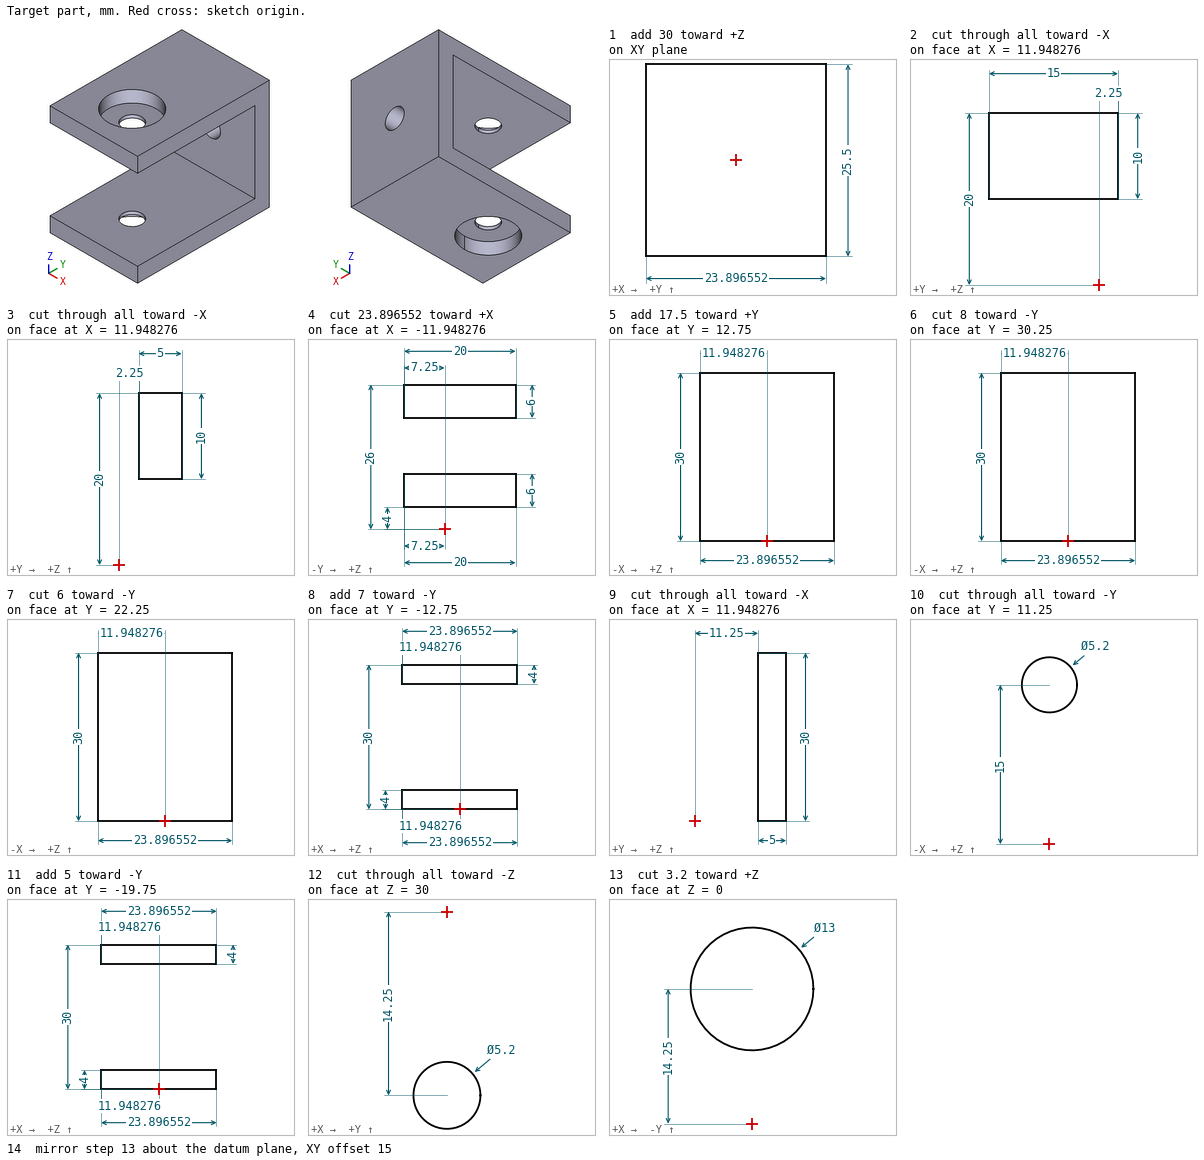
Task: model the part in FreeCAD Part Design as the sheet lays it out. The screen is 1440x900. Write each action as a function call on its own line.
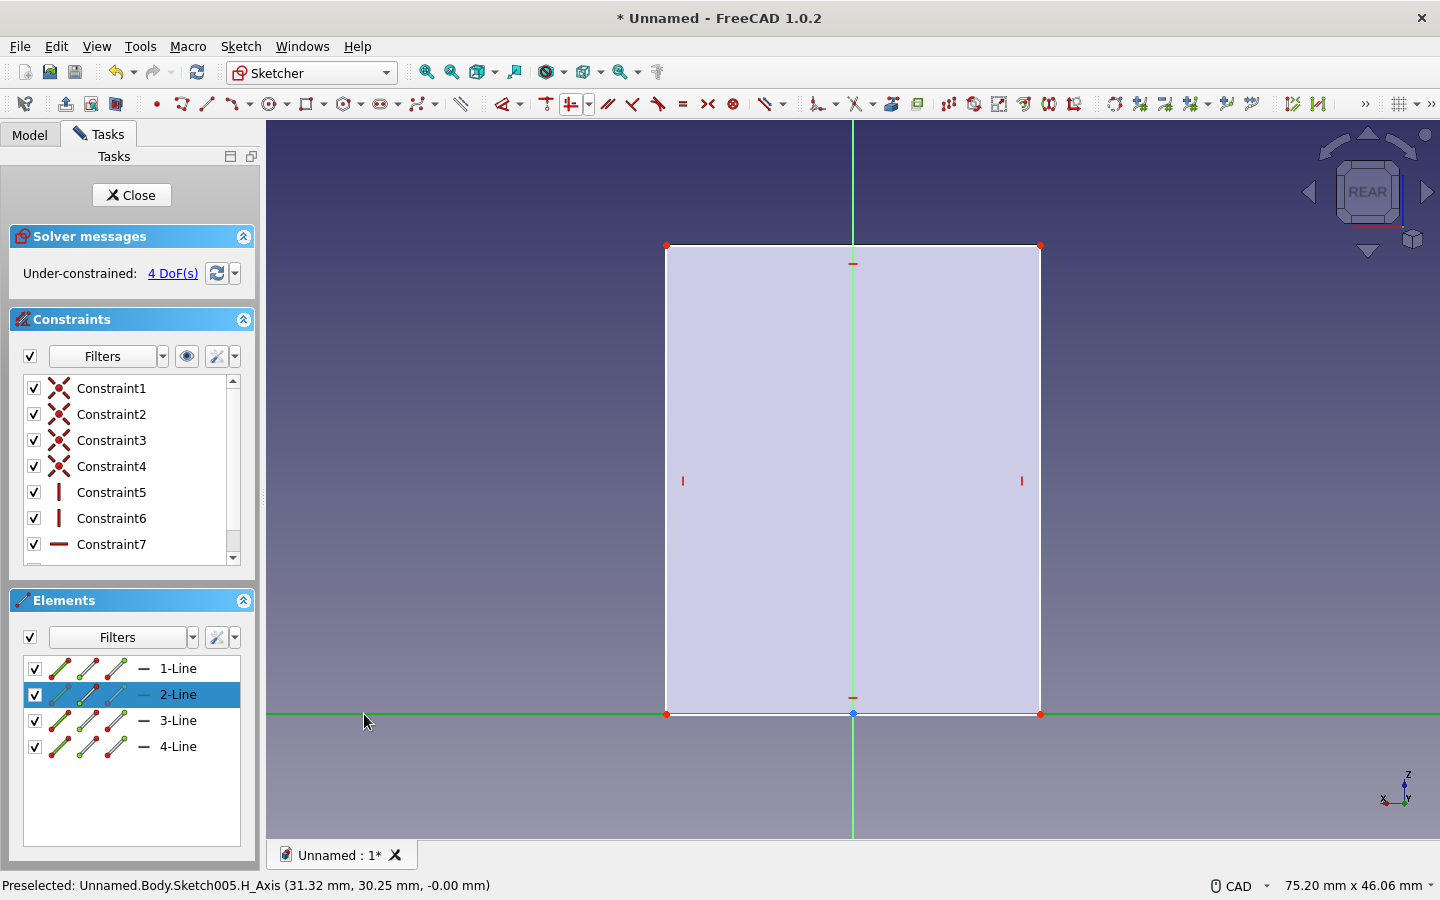
key(c)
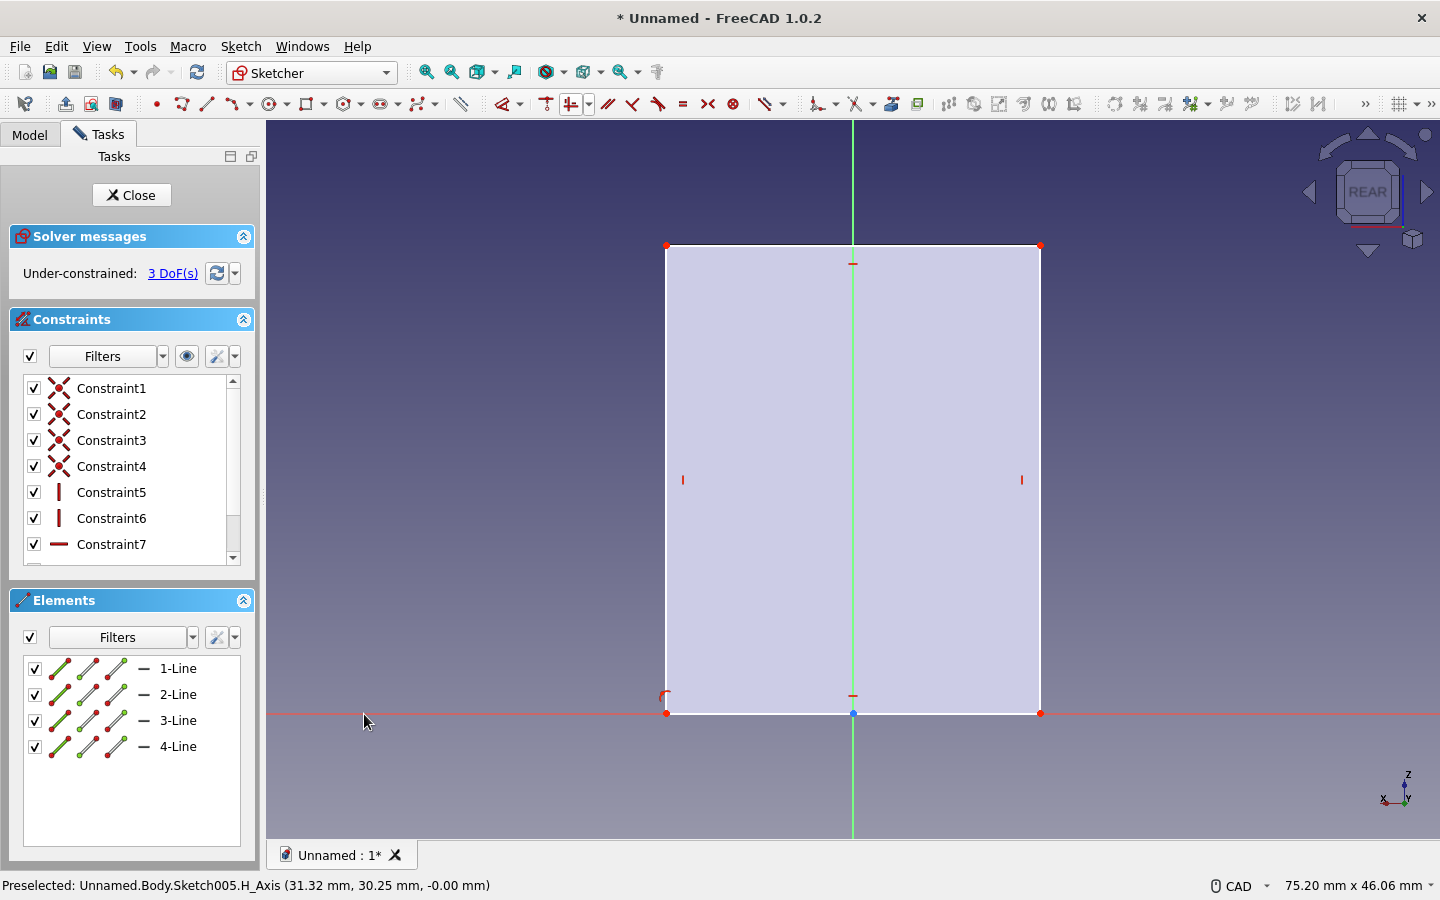
click(502, 104)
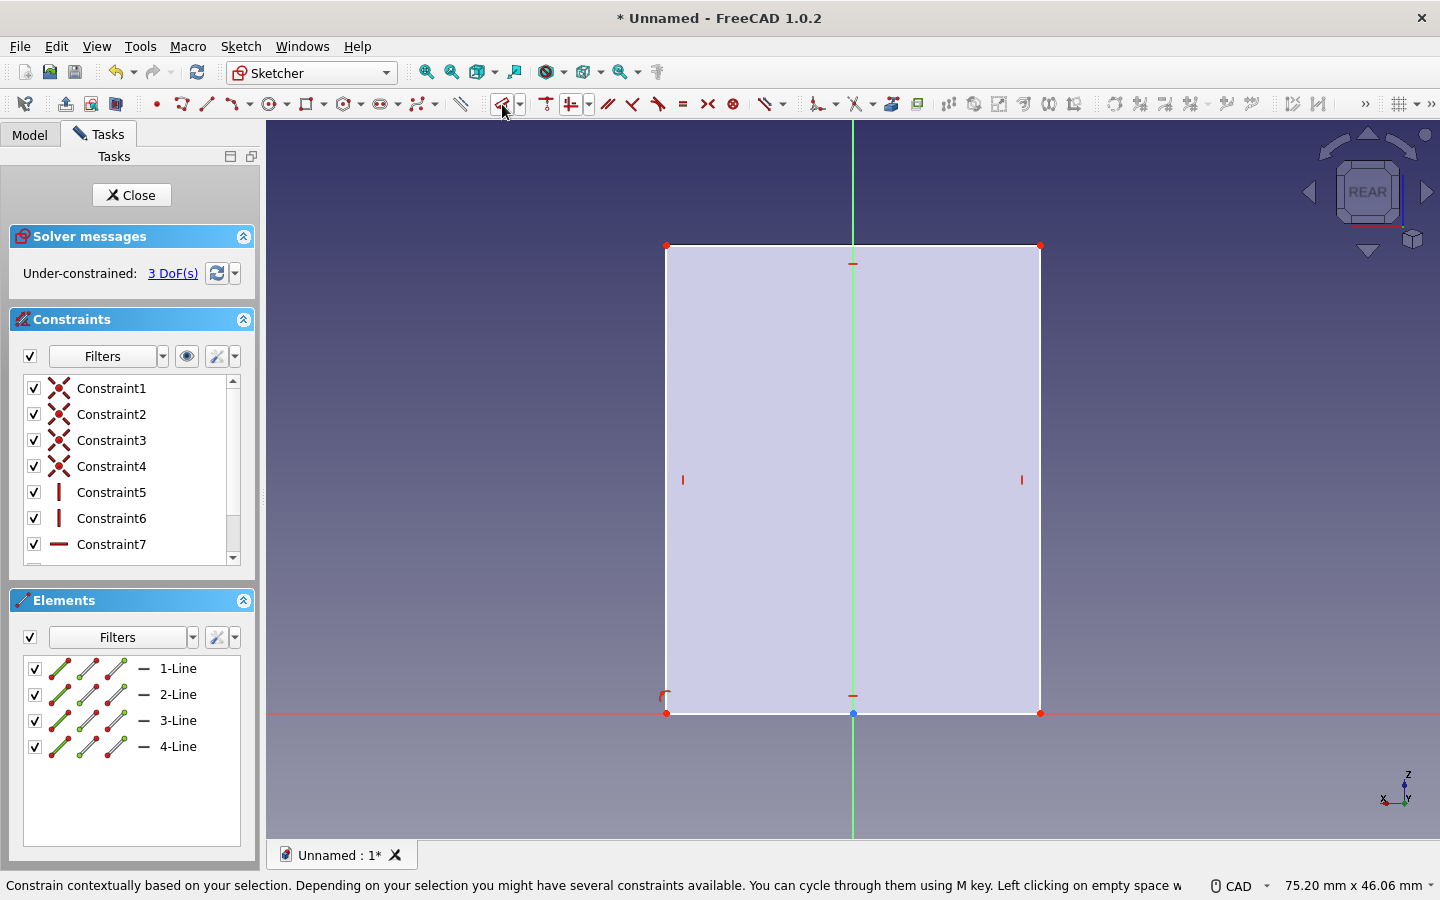
click(666, 386)
click(632, 480)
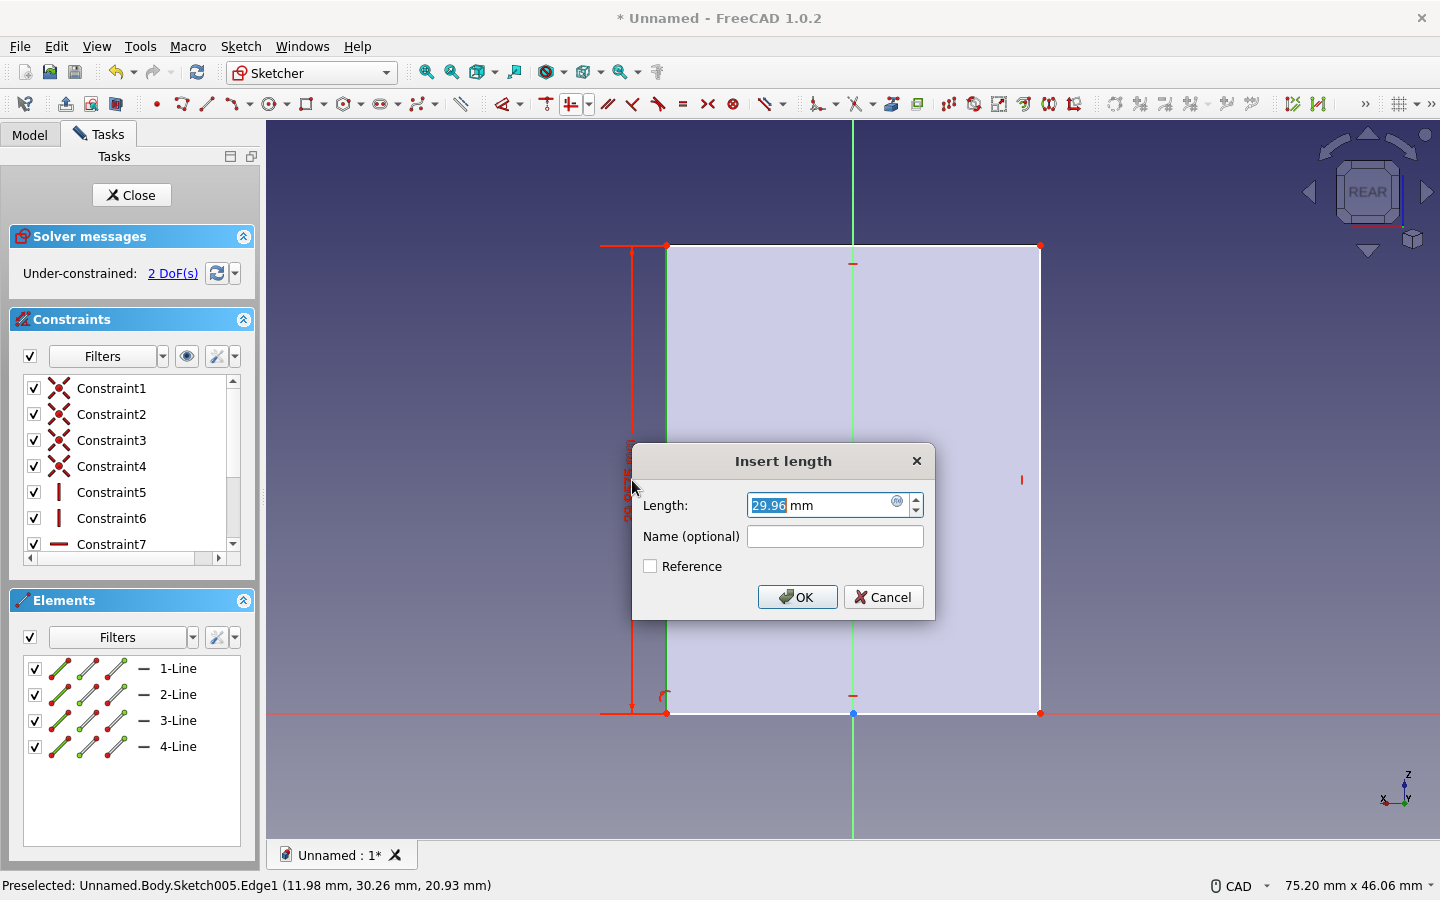
text(30)
key(Return)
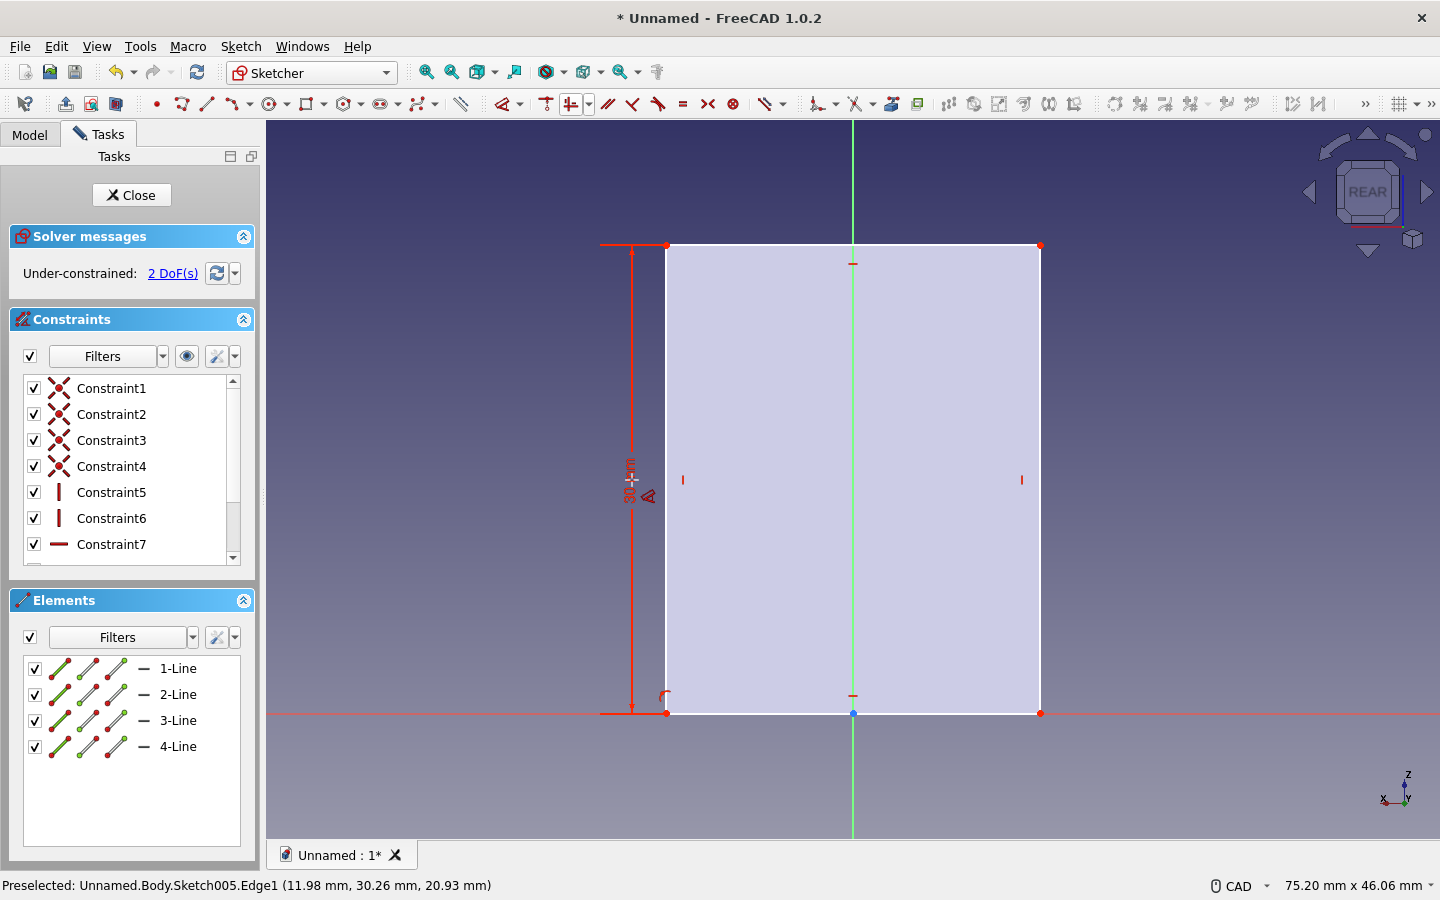
click(778, 714)
click(767, 748)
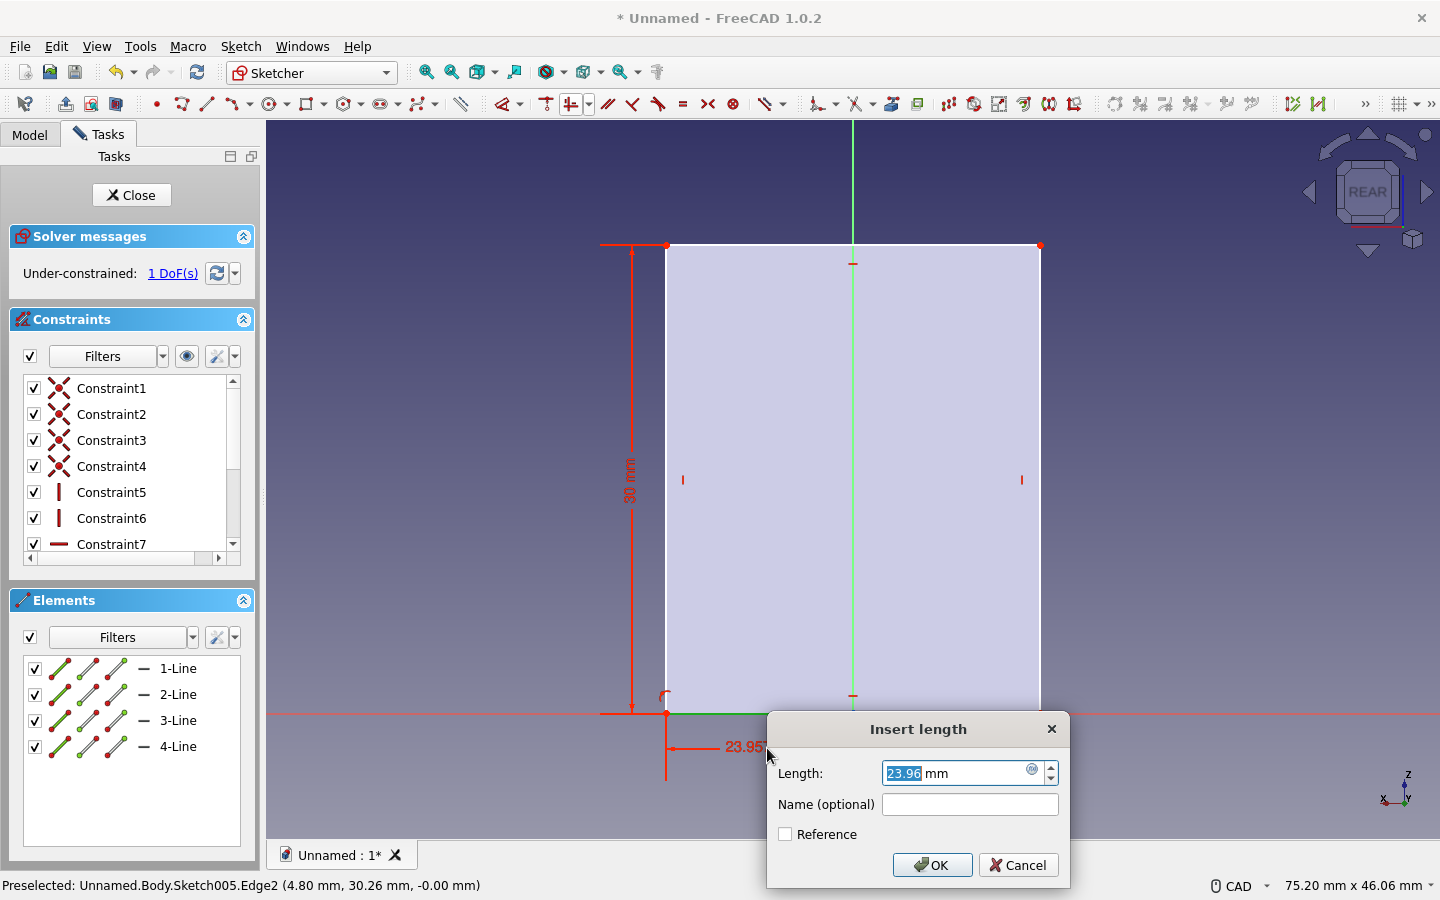
text(23.896552)
key(Return)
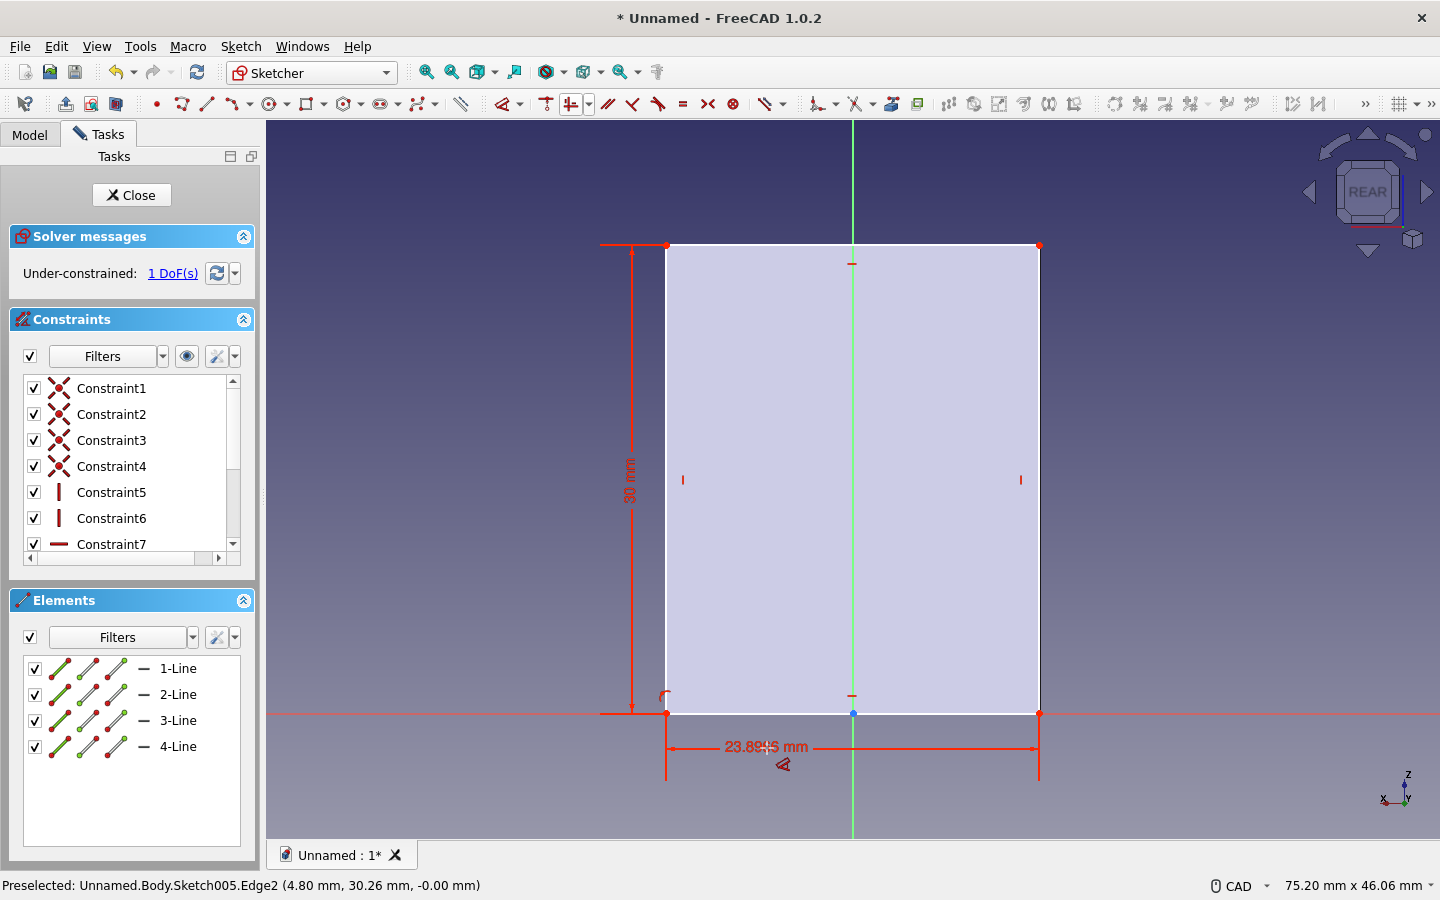
click(666, 245)
click(694, 748)